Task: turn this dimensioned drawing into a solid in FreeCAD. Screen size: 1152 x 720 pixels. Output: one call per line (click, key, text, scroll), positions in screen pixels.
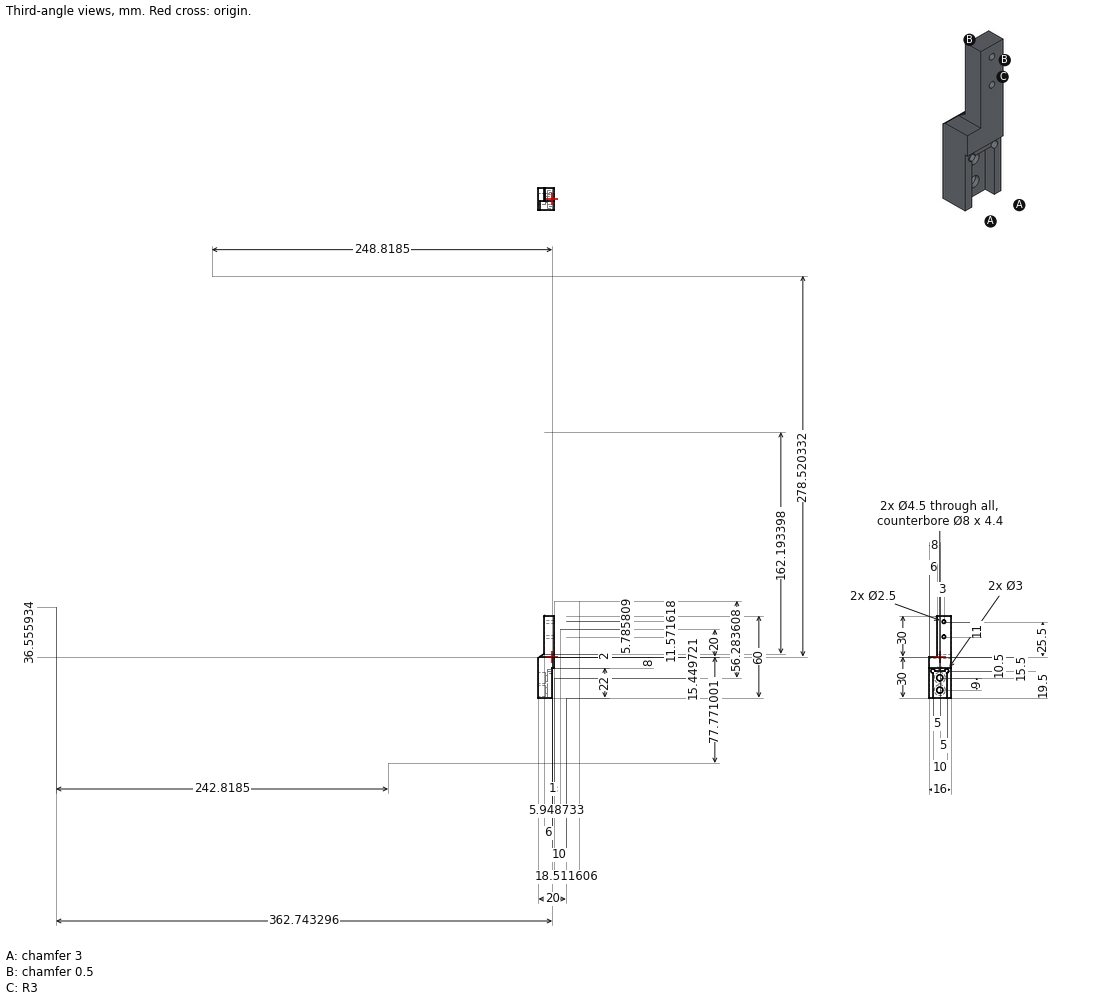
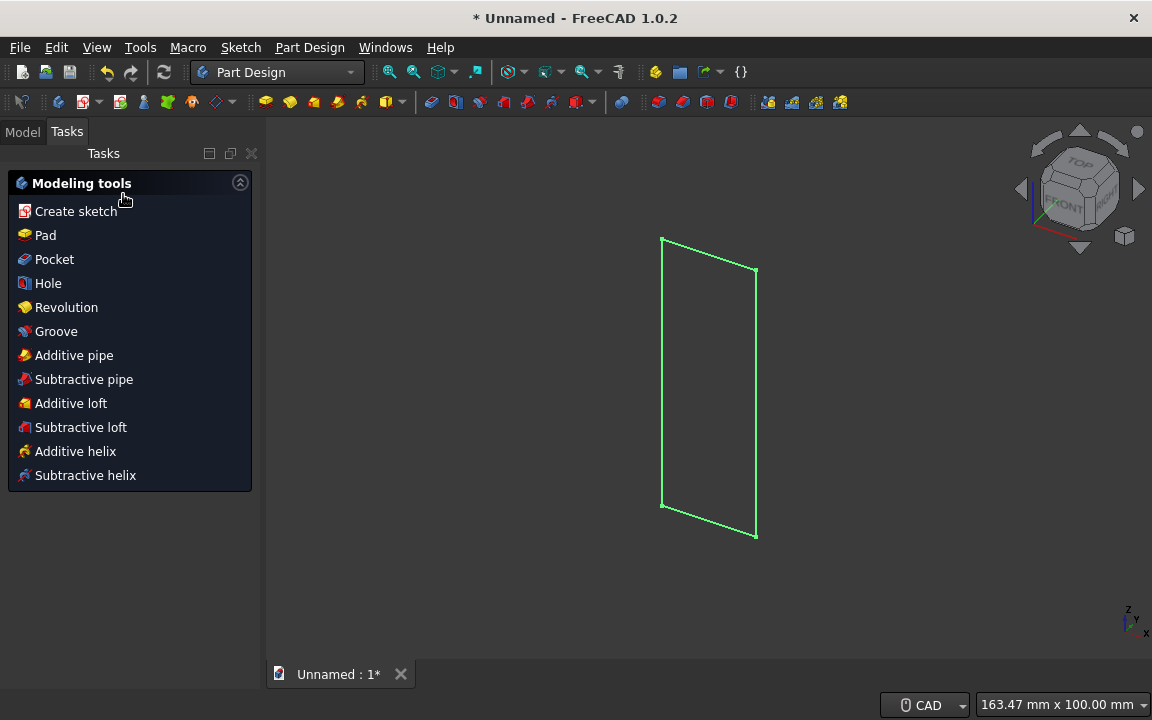
click(266, 102)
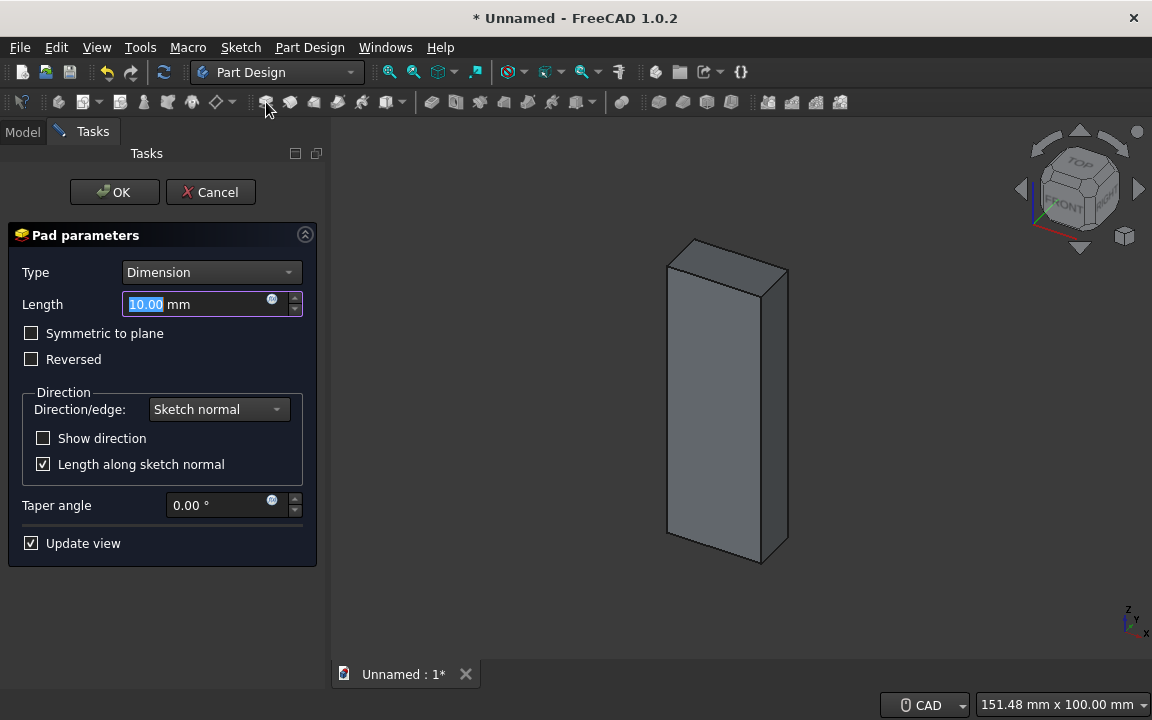
text(16)
key(Tab)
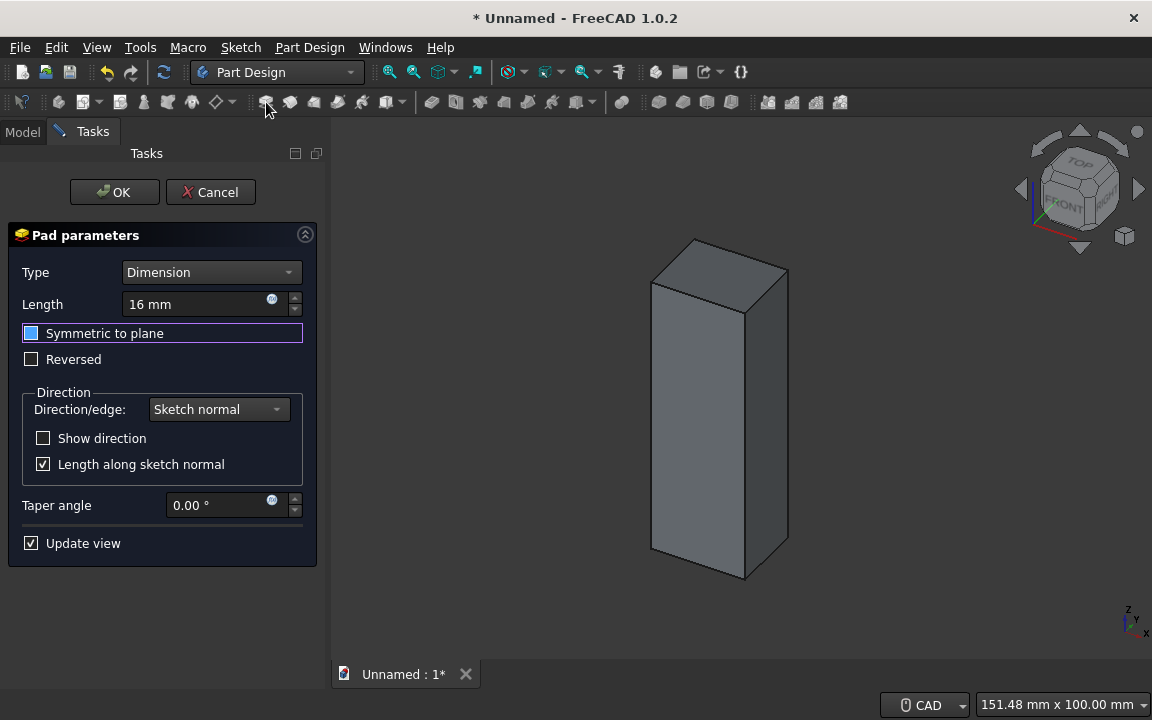
click(30, 333)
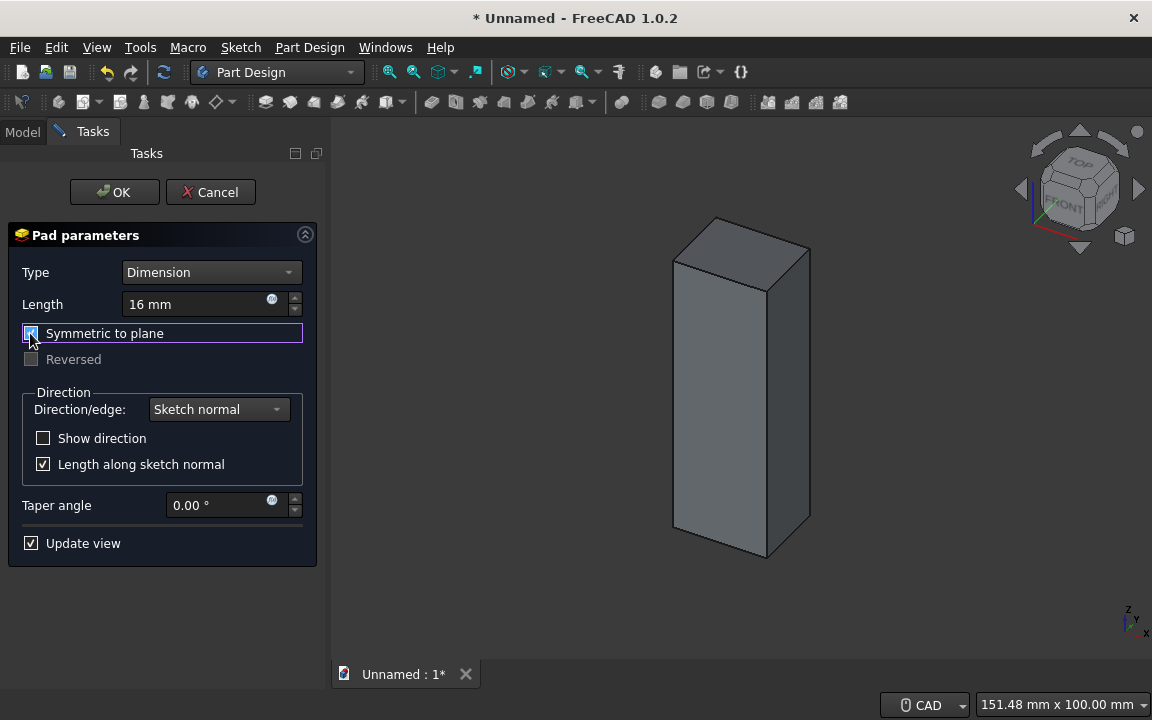
click(115, 192)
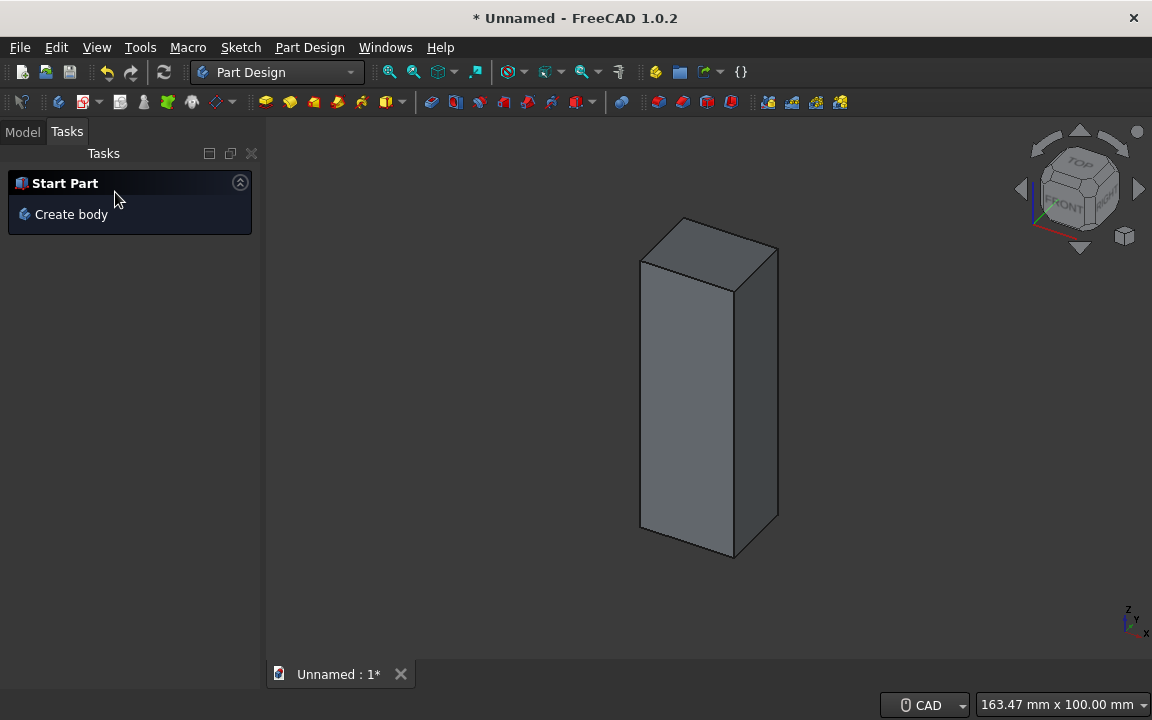
click(756, 326)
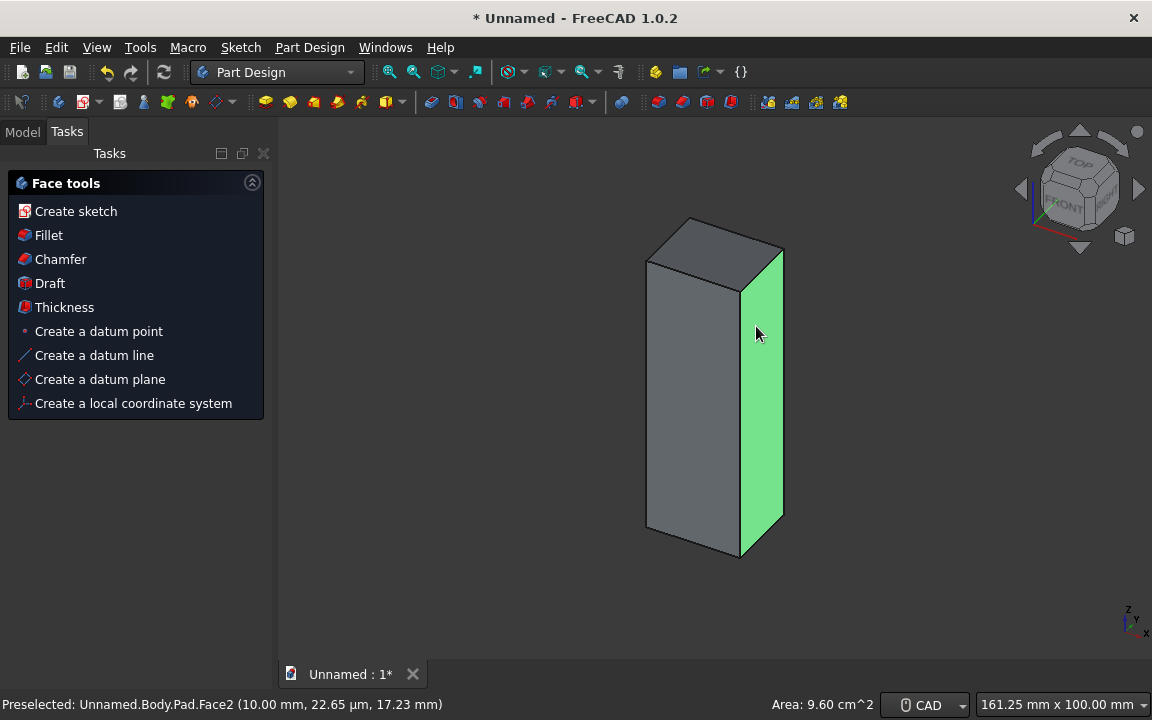
click(84, 102)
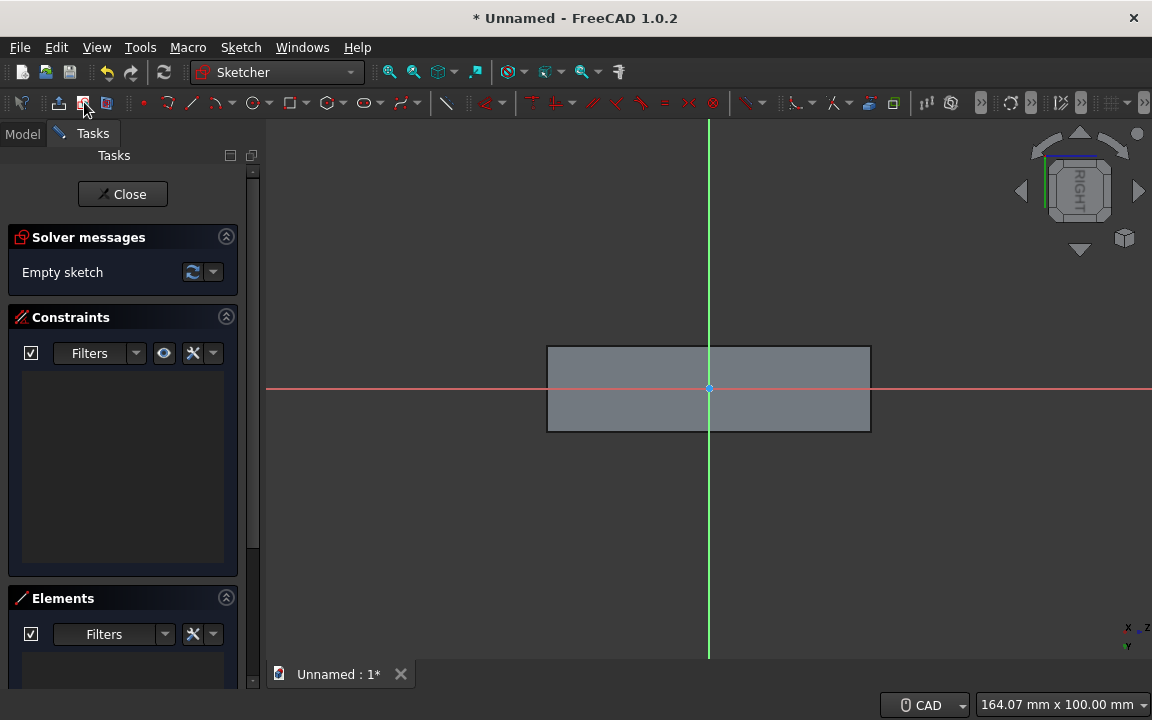
scroll(623, 389, up, 6)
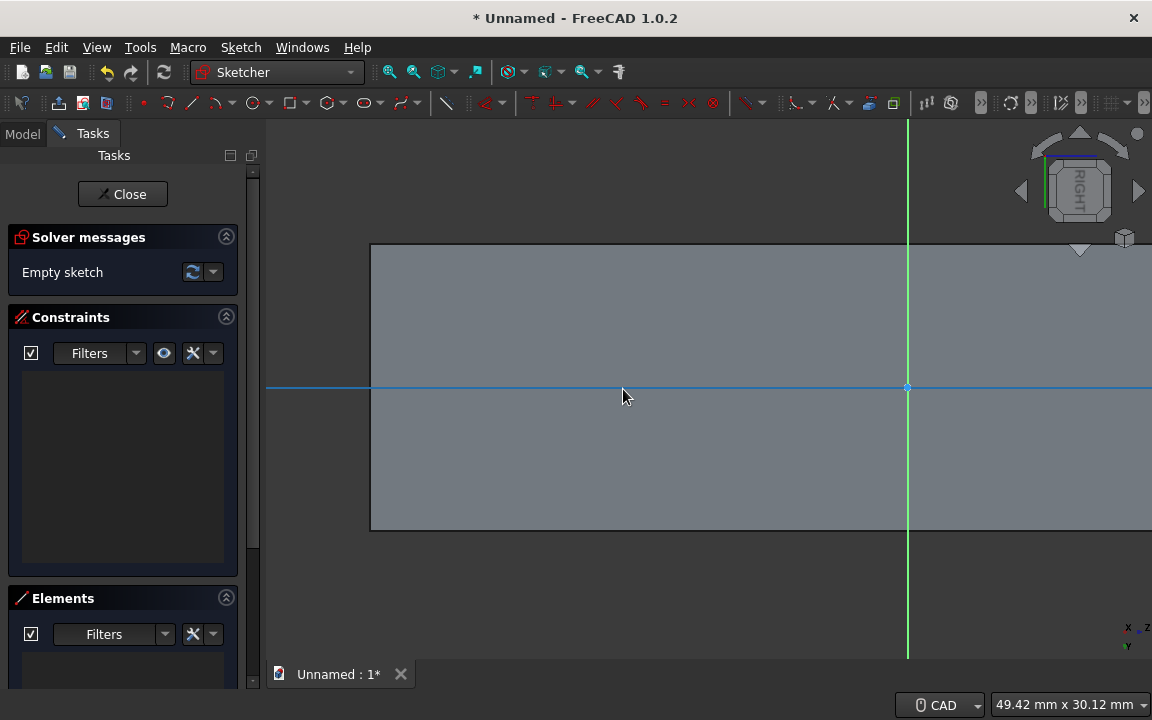
click(290, 104)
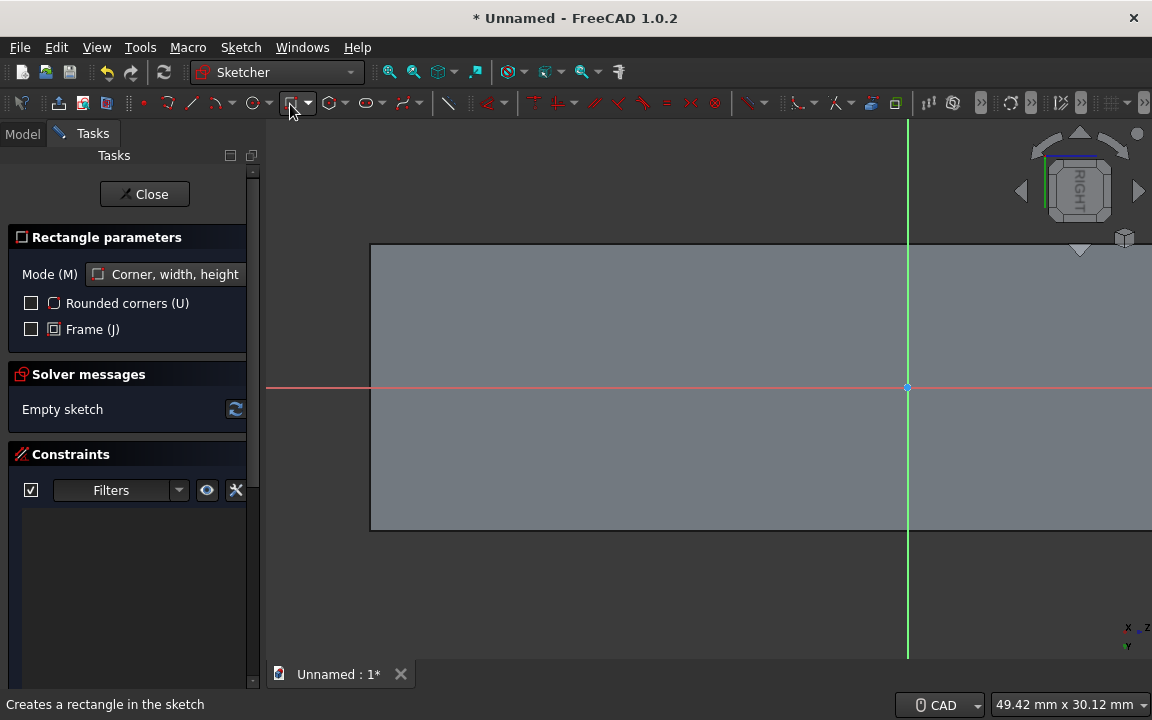
click(370, 298)
click(719, 477)
key(Escape)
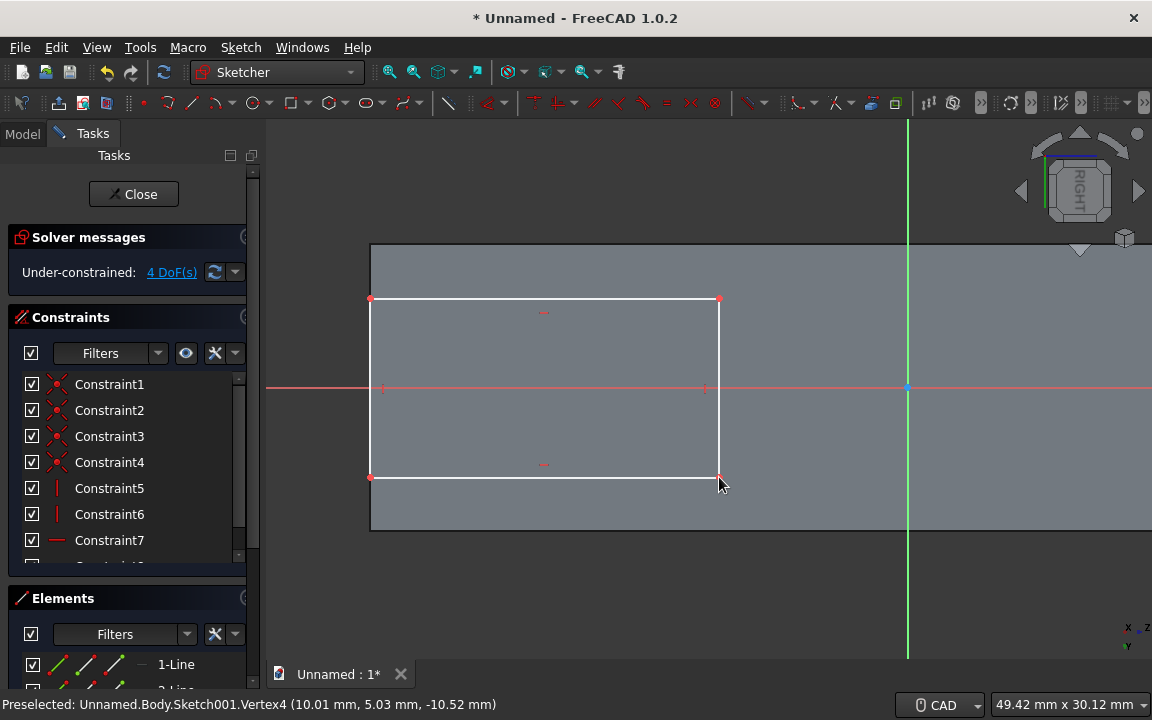
click(488, 104)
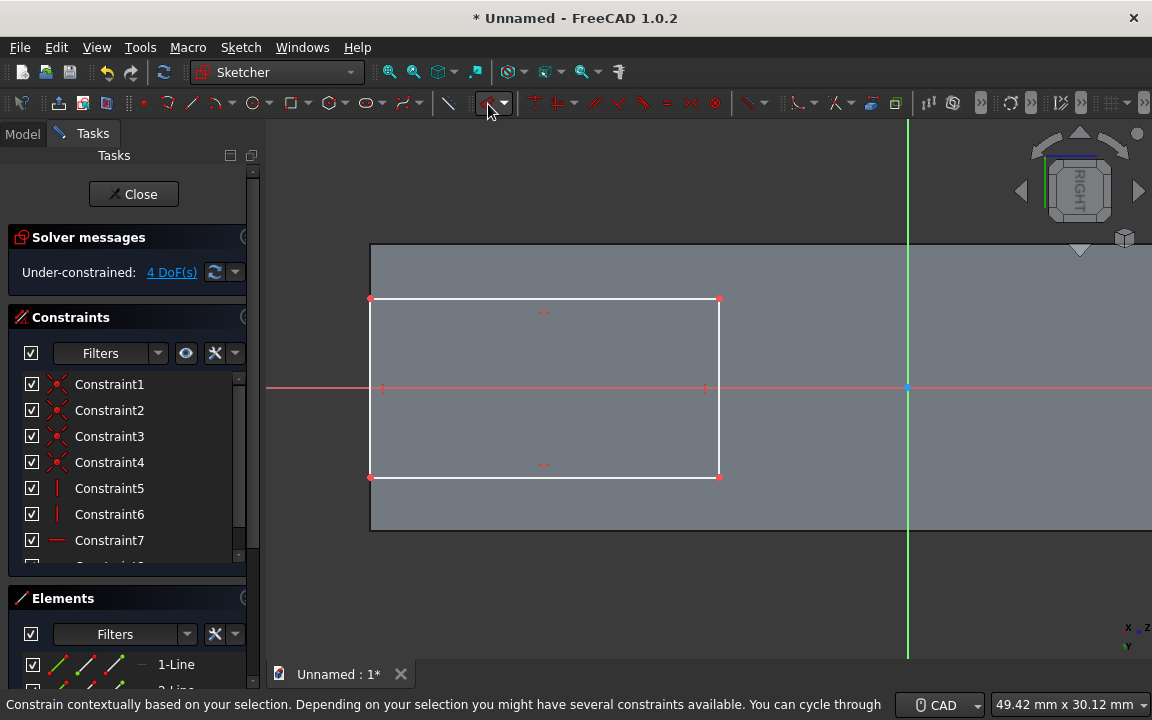
click(370, 353)
click(336, 347)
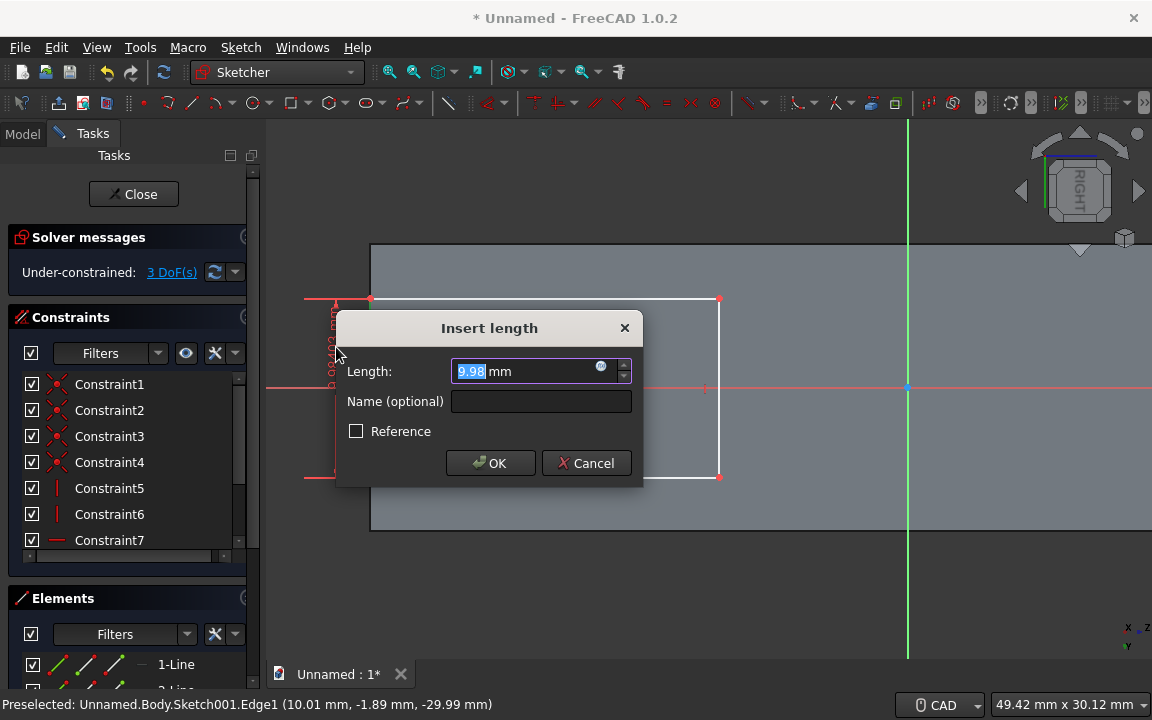
text(10)
key(Return)